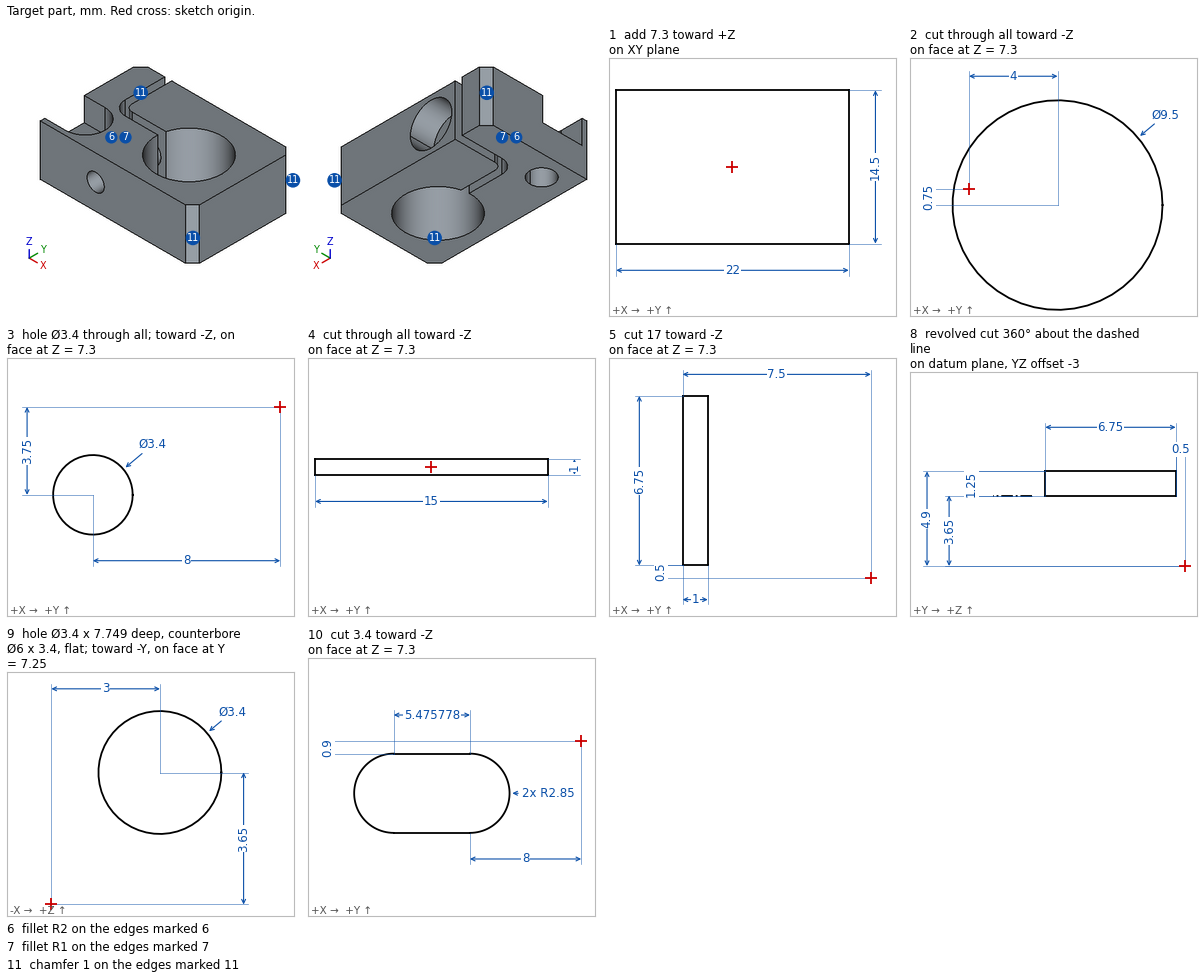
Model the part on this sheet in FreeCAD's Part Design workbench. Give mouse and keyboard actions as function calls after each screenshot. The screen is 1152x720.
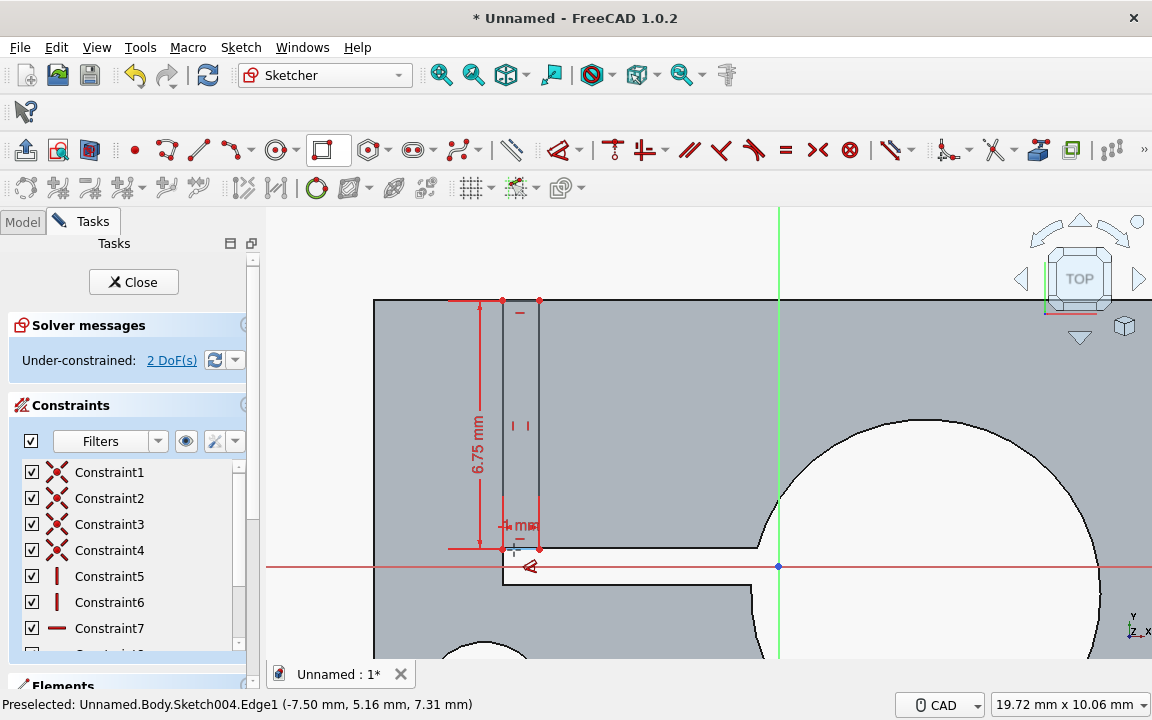
click(503, 301)
click(641, 601)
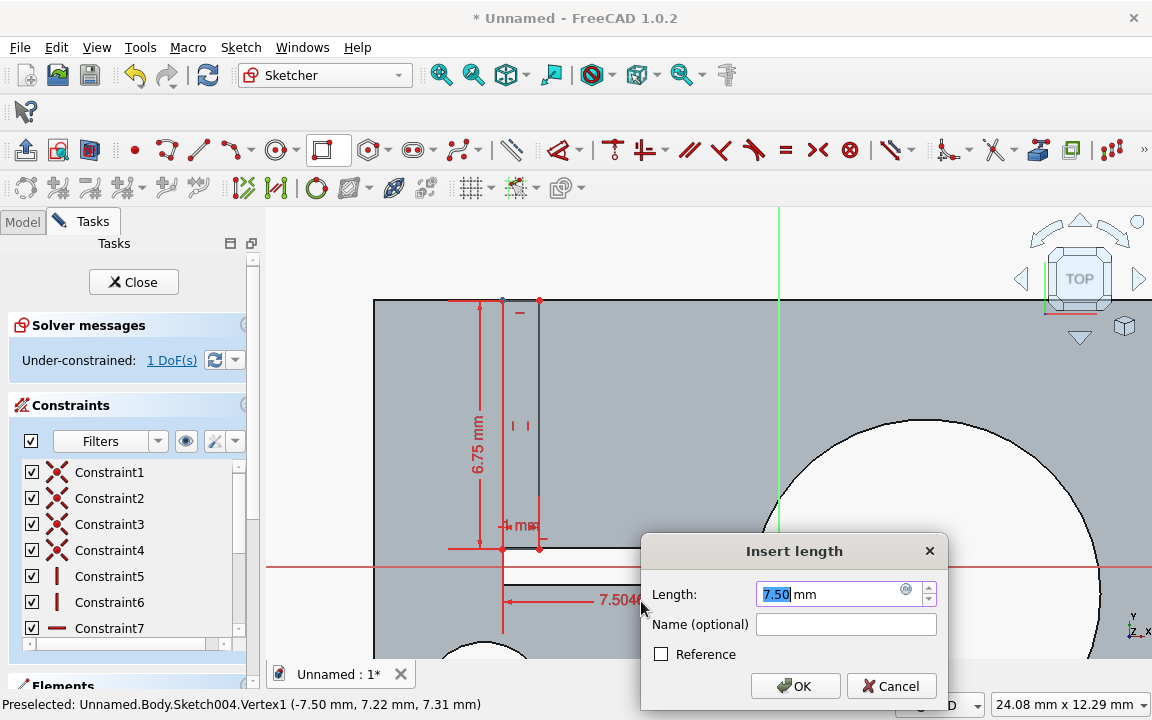
text(7.5)
key(Return)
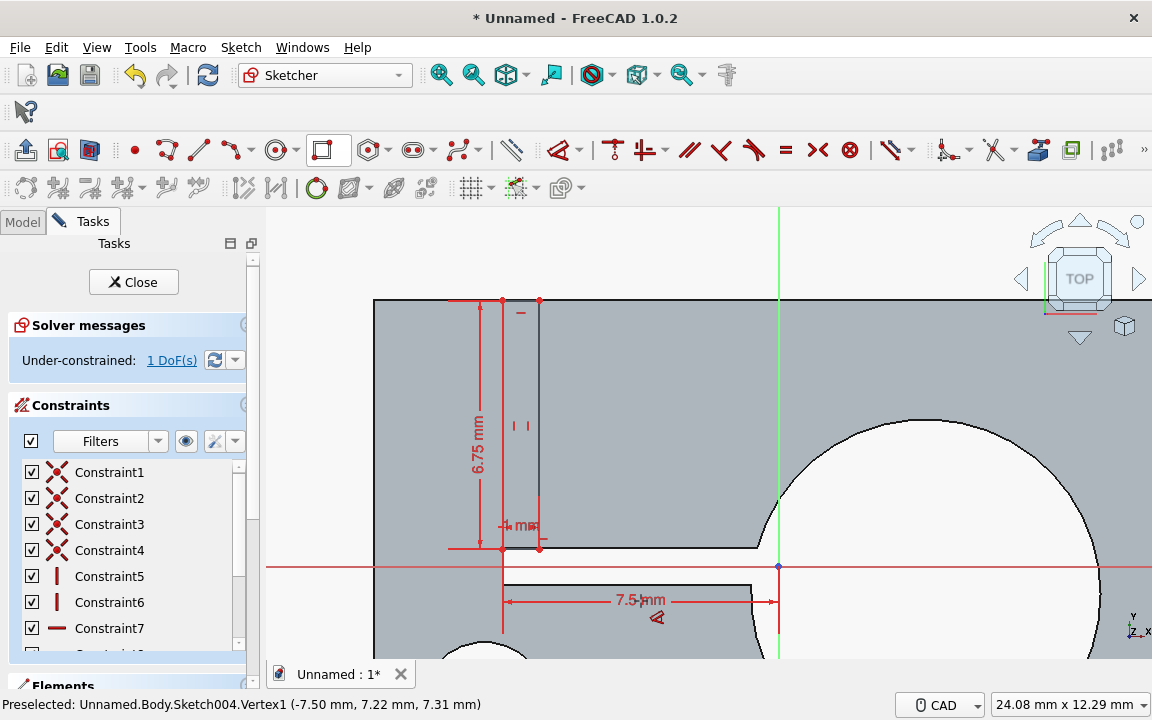
scroll(503, 549, up, 4)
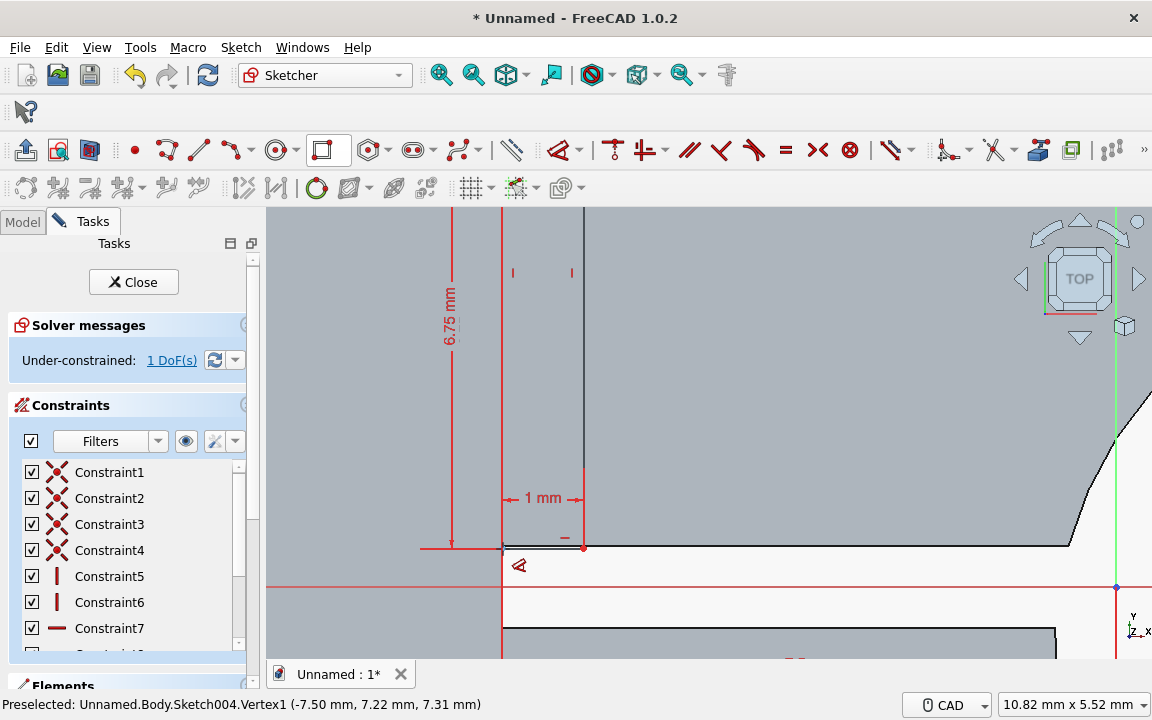
click(502, 549)
click(468, 568)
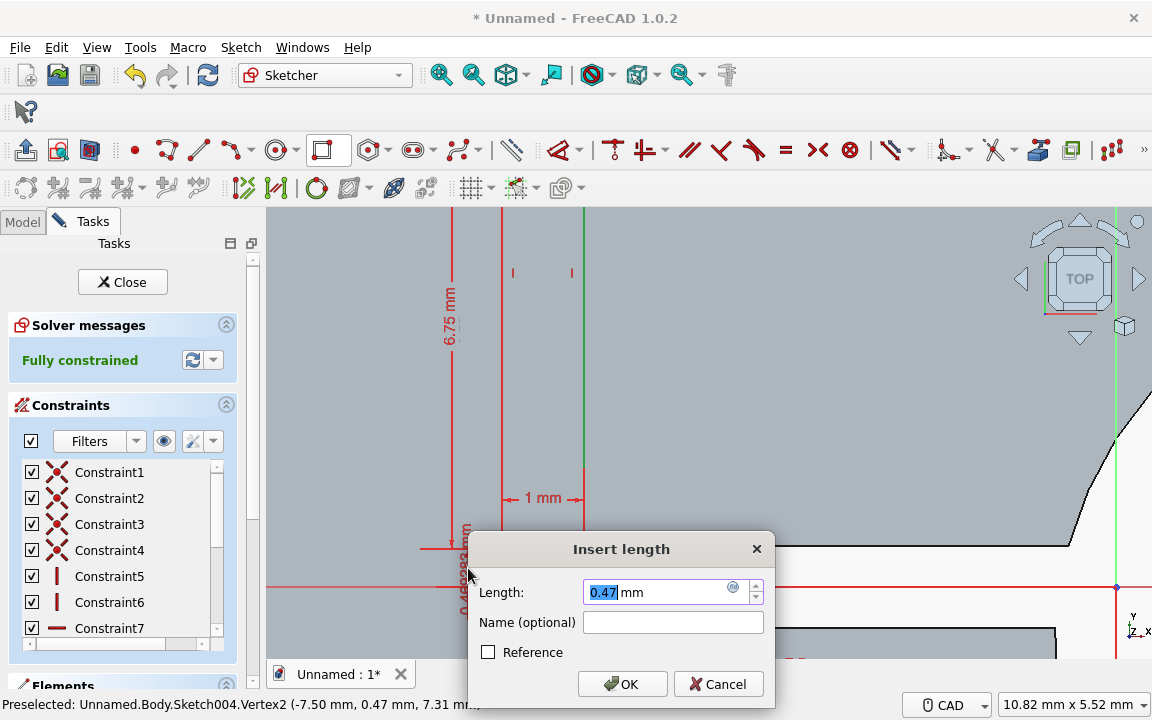
text(0.5)
key(Return)
key(Escape)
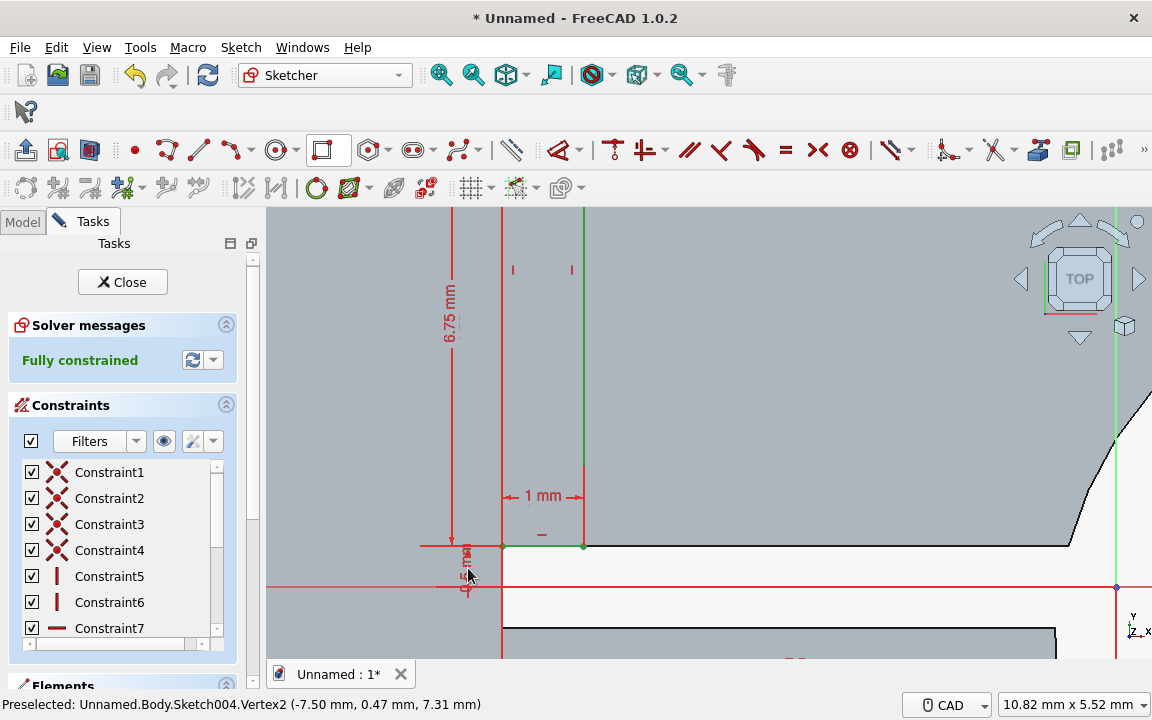
click(123, 282)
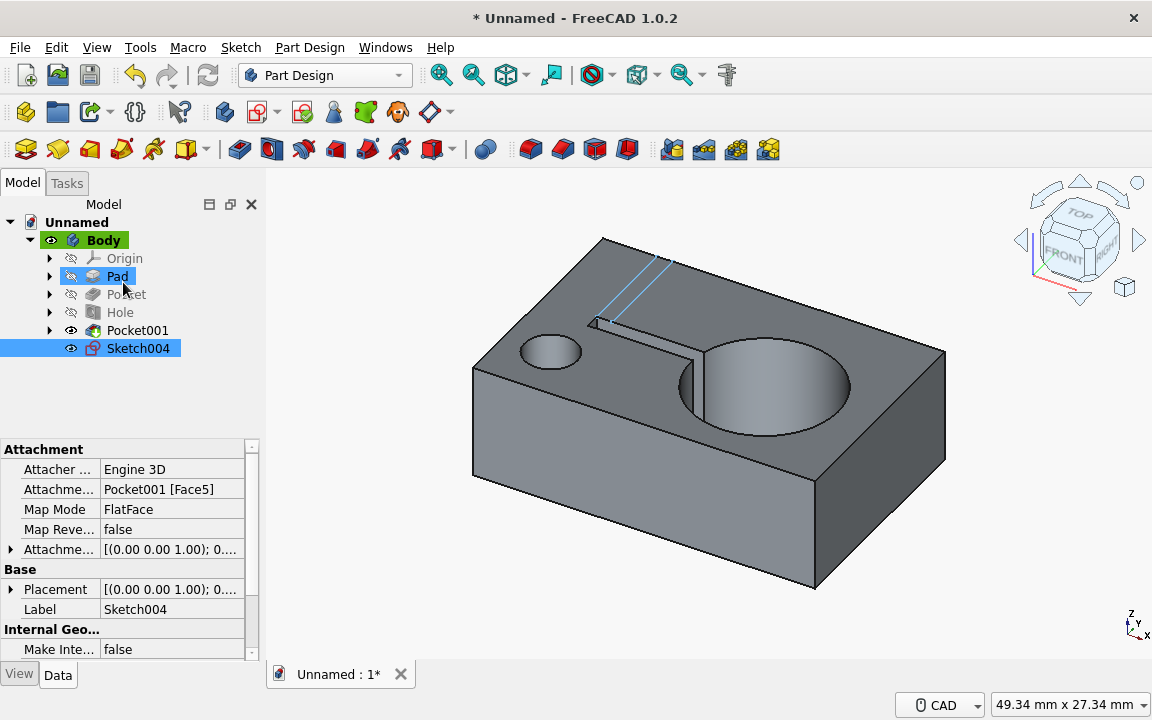
click(240, 150)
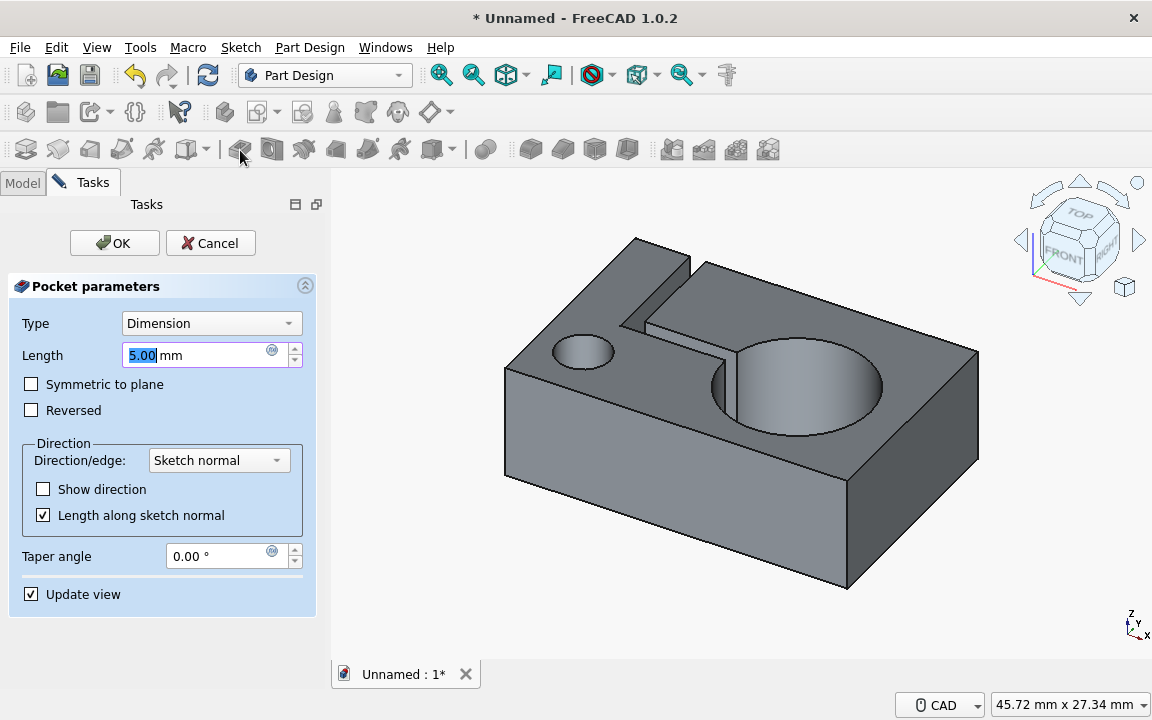
text(17)
key(Tab)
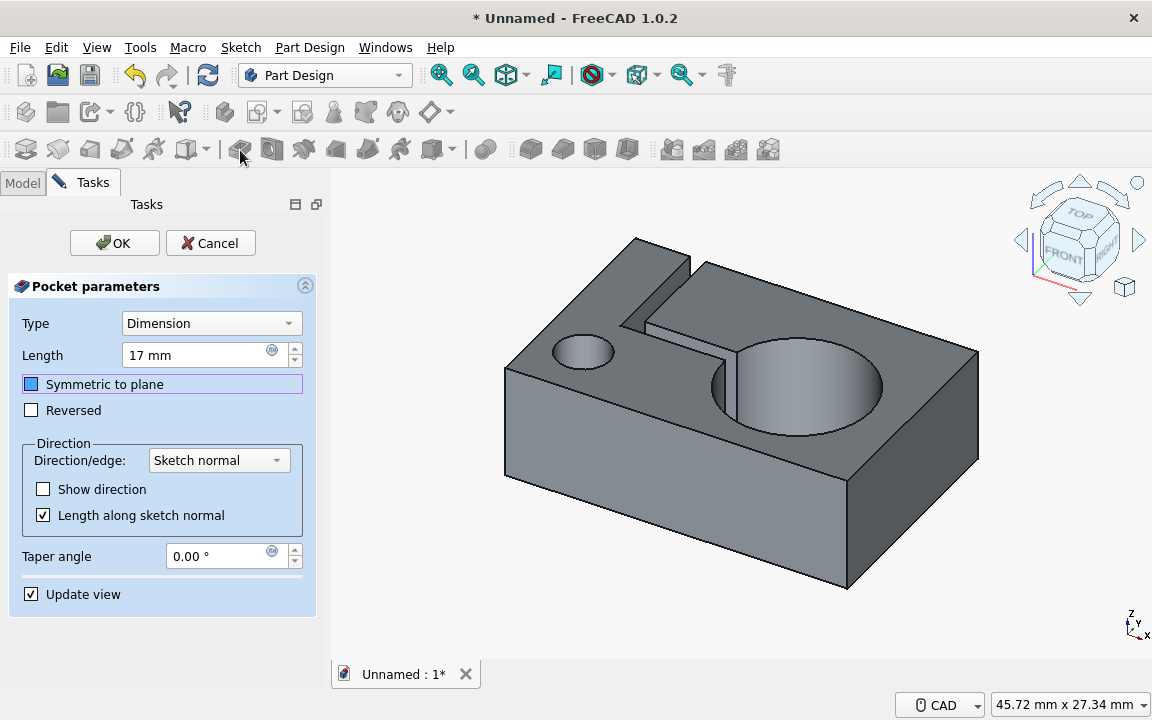
click(115, 243)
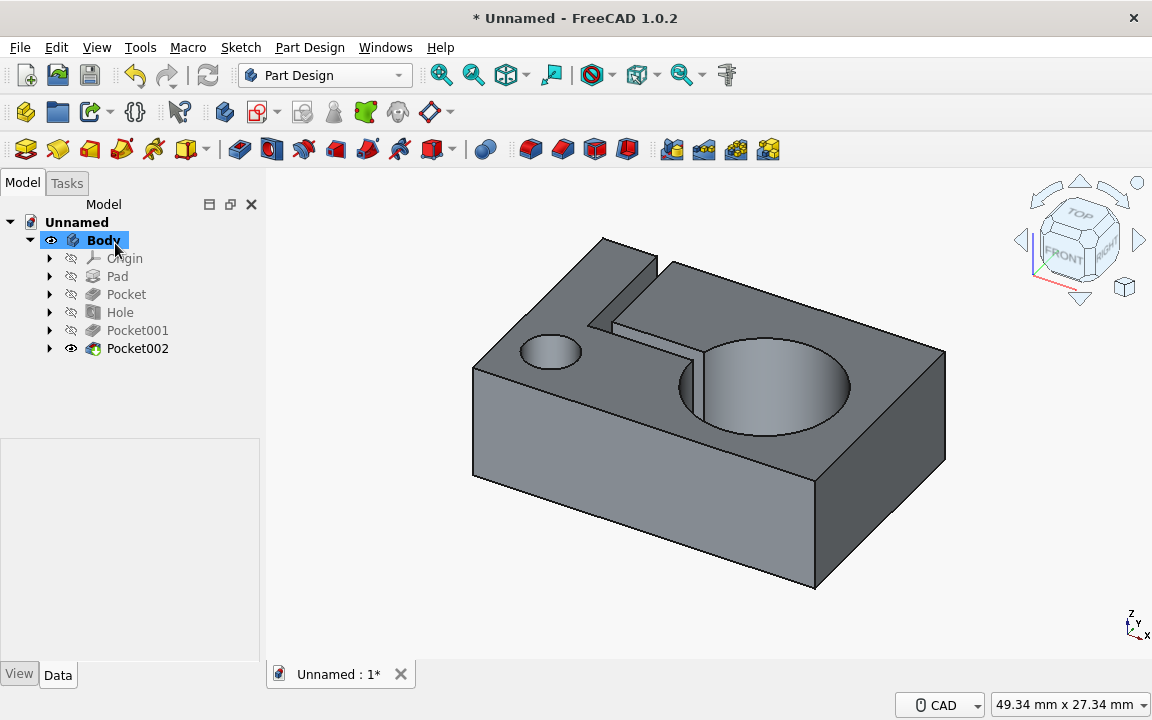
key(0)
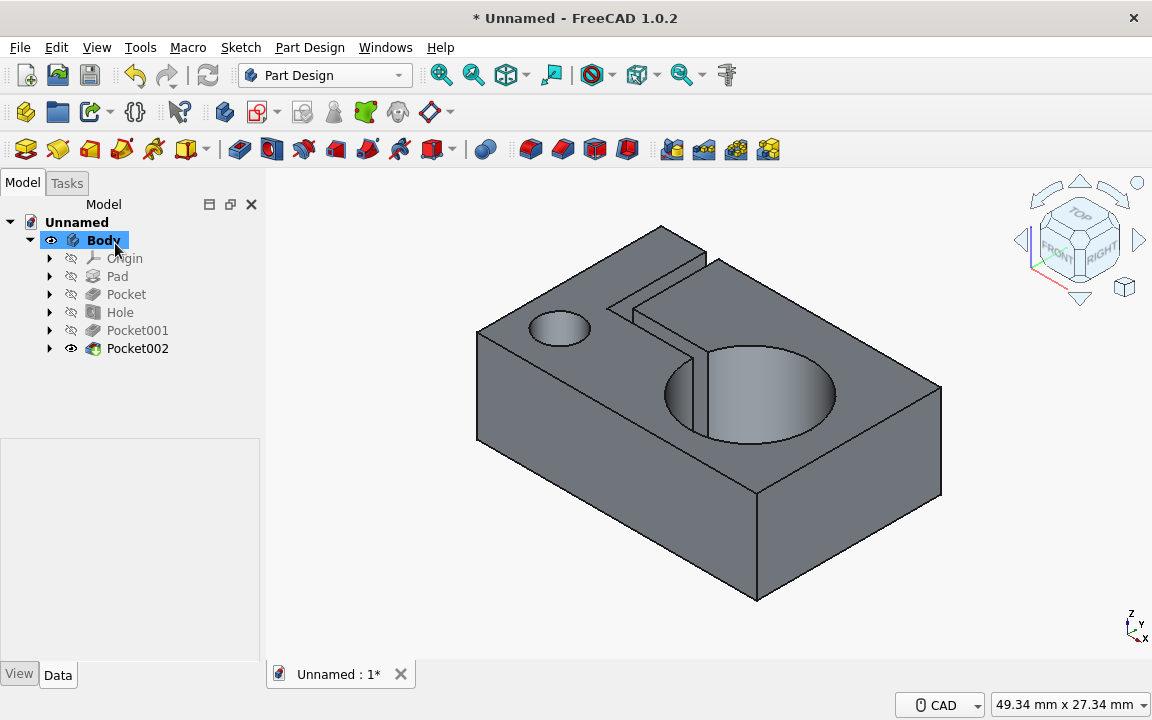
key(2)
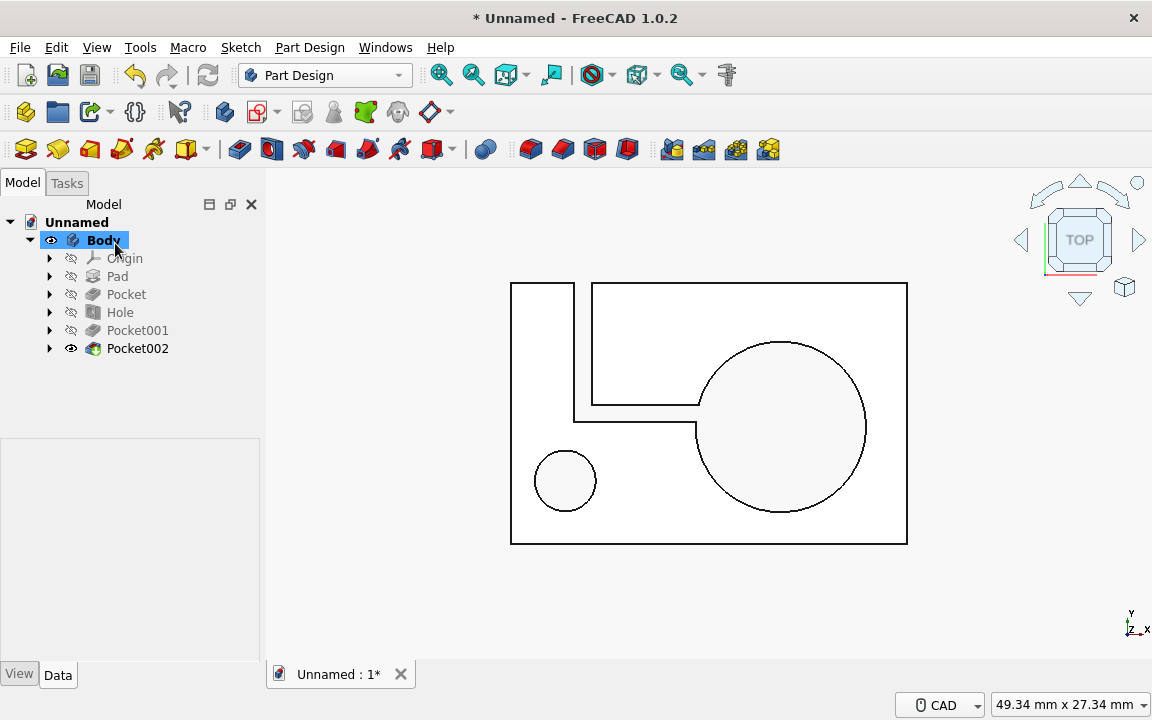
key(1)